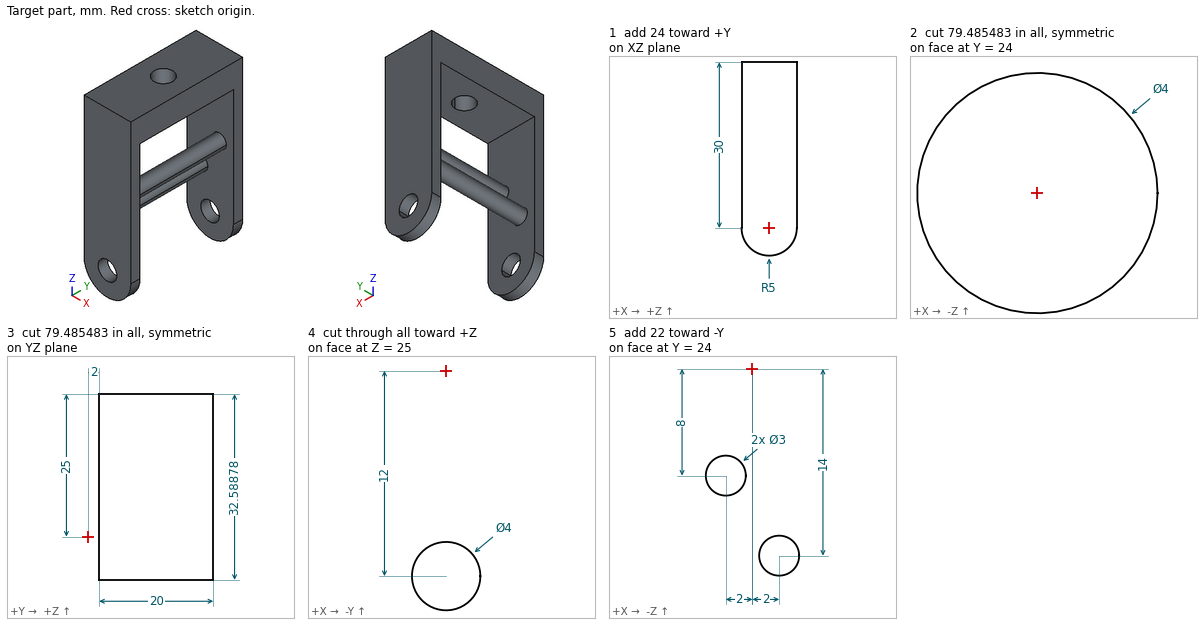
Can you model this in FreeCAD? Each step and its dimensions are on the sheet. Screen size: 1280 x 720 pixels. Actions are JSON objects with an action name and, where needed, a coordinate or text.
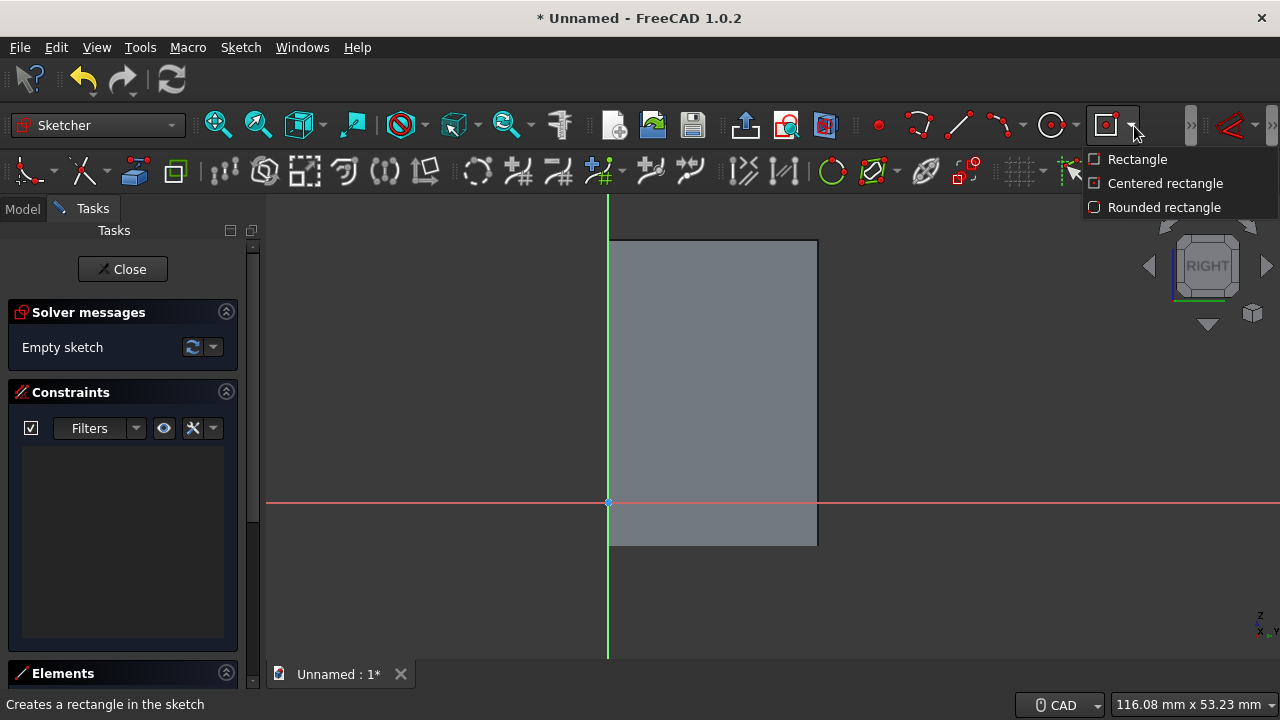
{"action": "left_click", "coordinate": [1180, 159]}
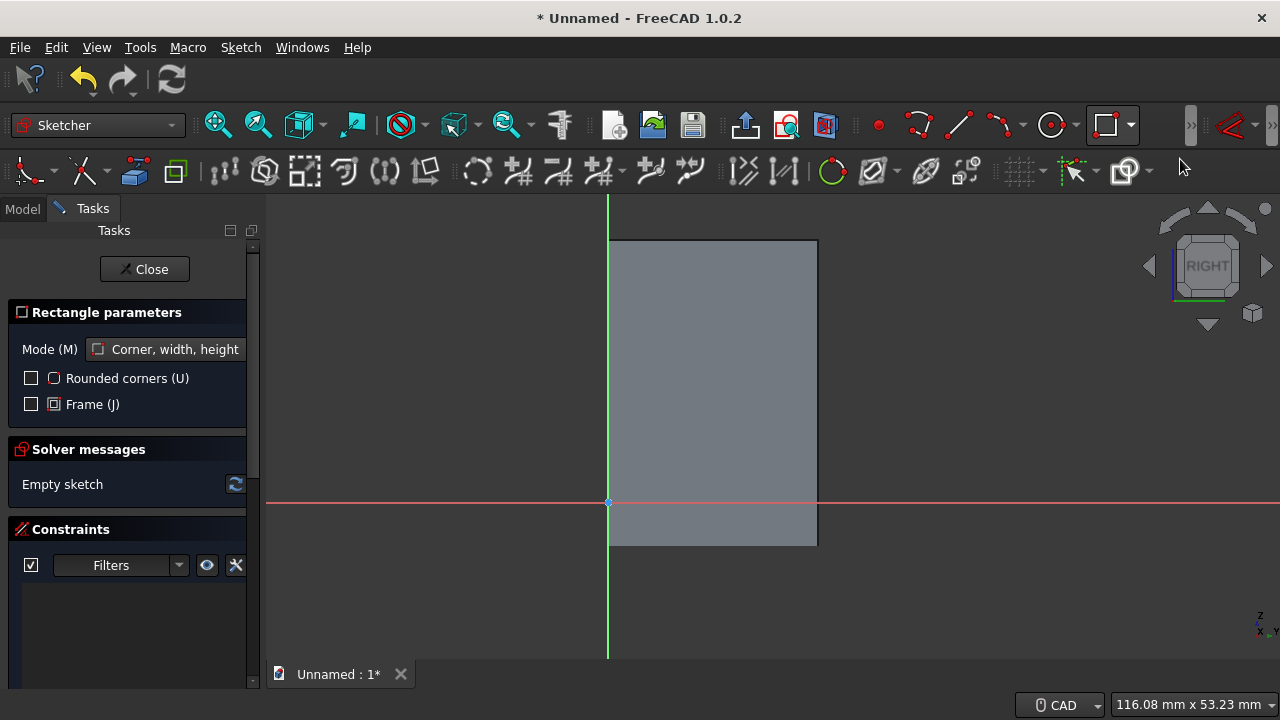
{"action": "left_click", "coordinate": [626, 284]}
{"action": "mouse_move", "coordinate": [801, 569]}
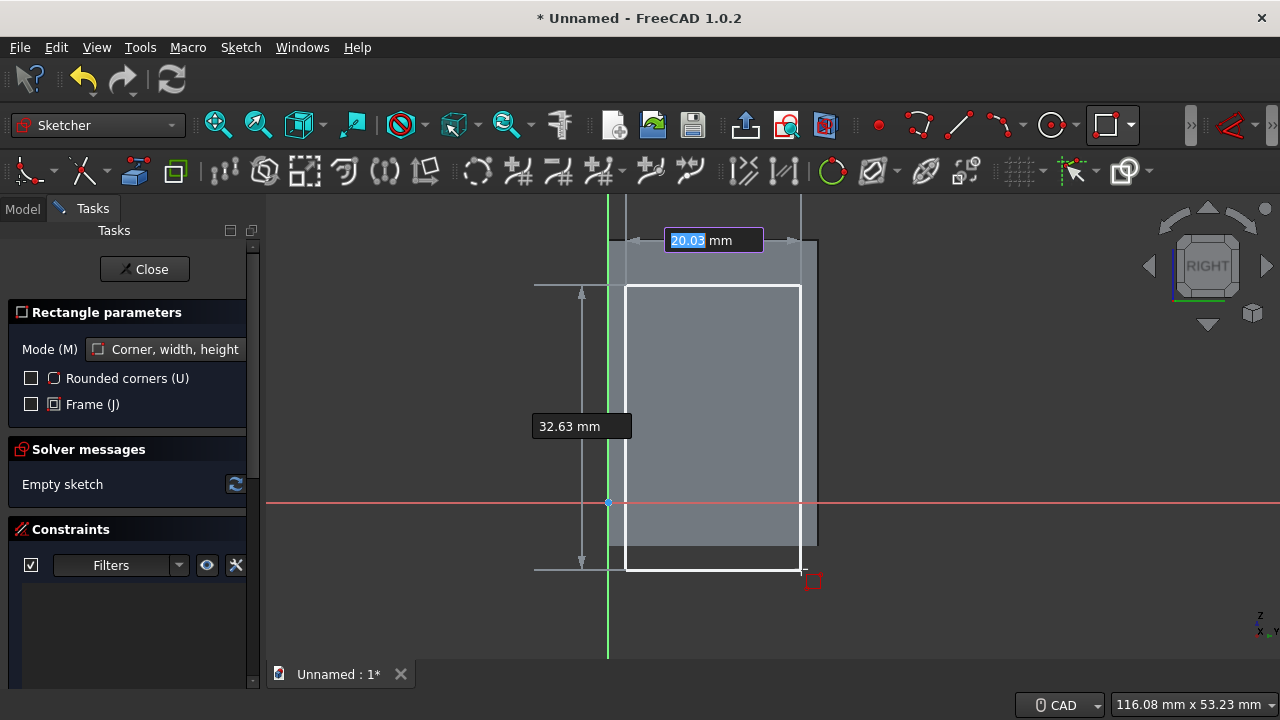
{"action": "type", "text": "20"}
{"action": "key", "text": "Tab"}
{"action": "type", "text": "32.58878"}
{"action": "key", "text": "Return"}
{"action": "key", "text": "Escape"}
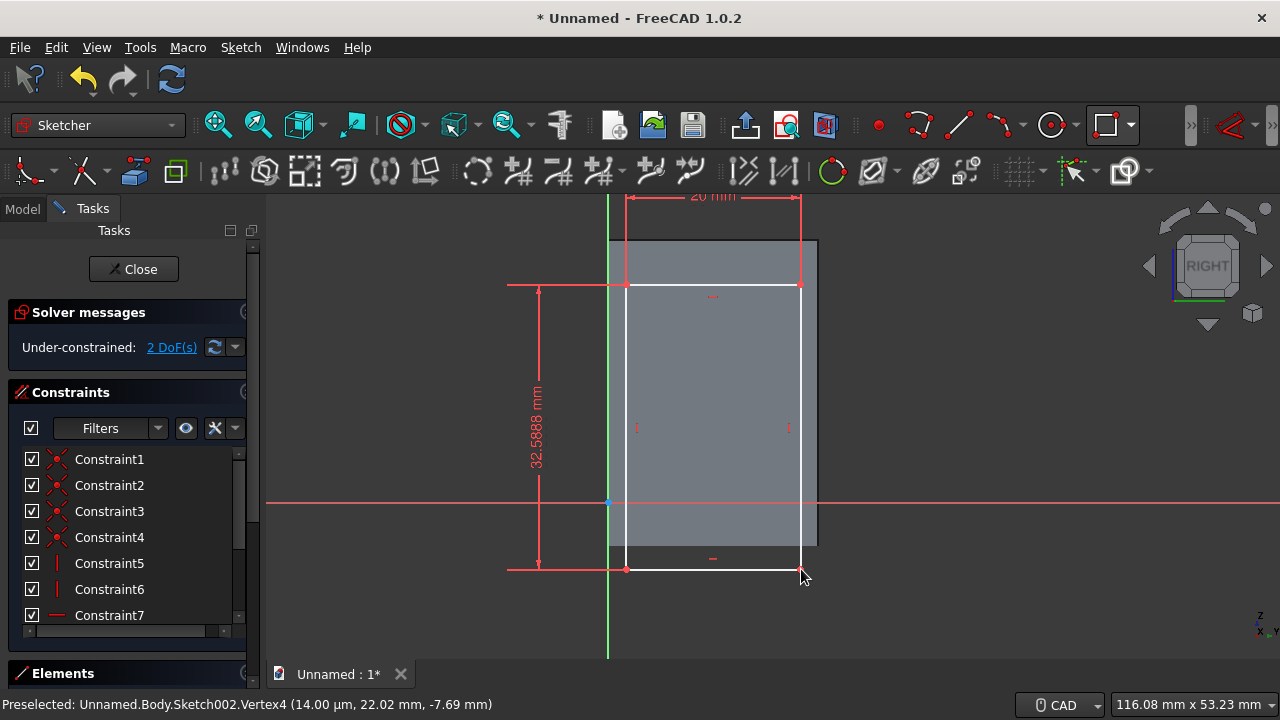
{"action": "left_click", "coordinate": [1230, 126]}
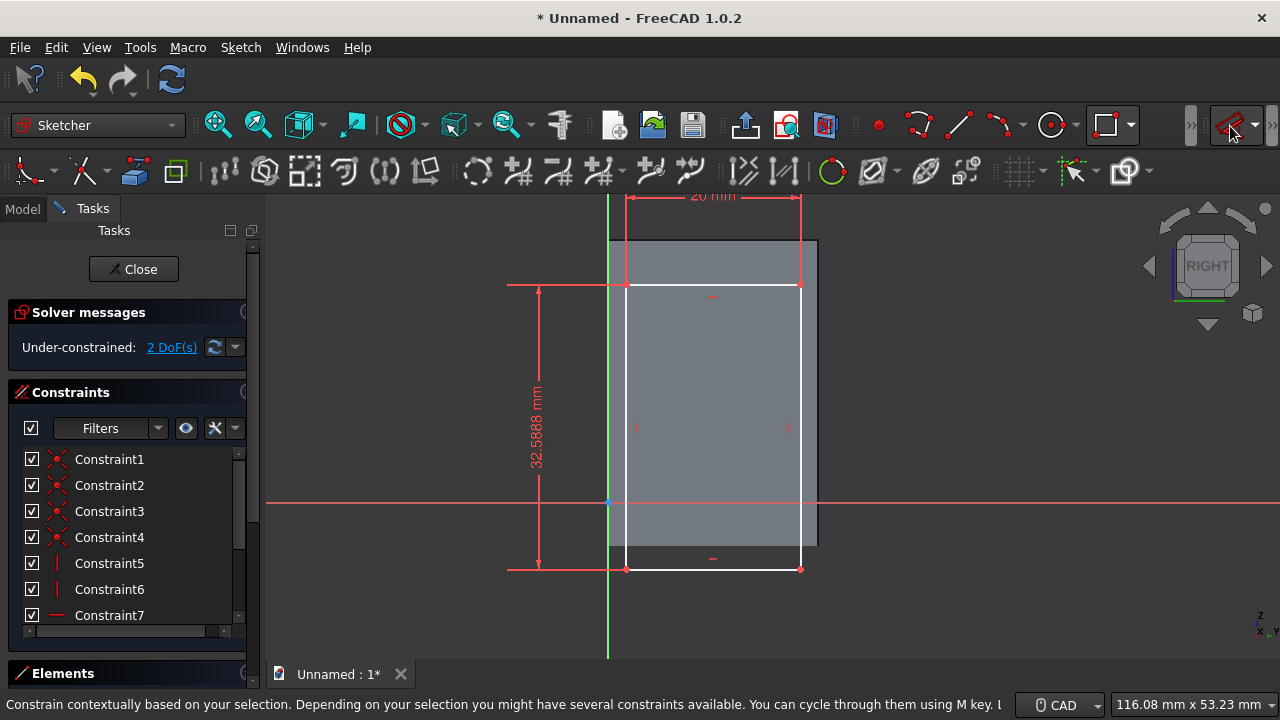
{"action": "scroll", "coordinate": [626, 285], "scroll_direction": "up", "scroll_amount": 5}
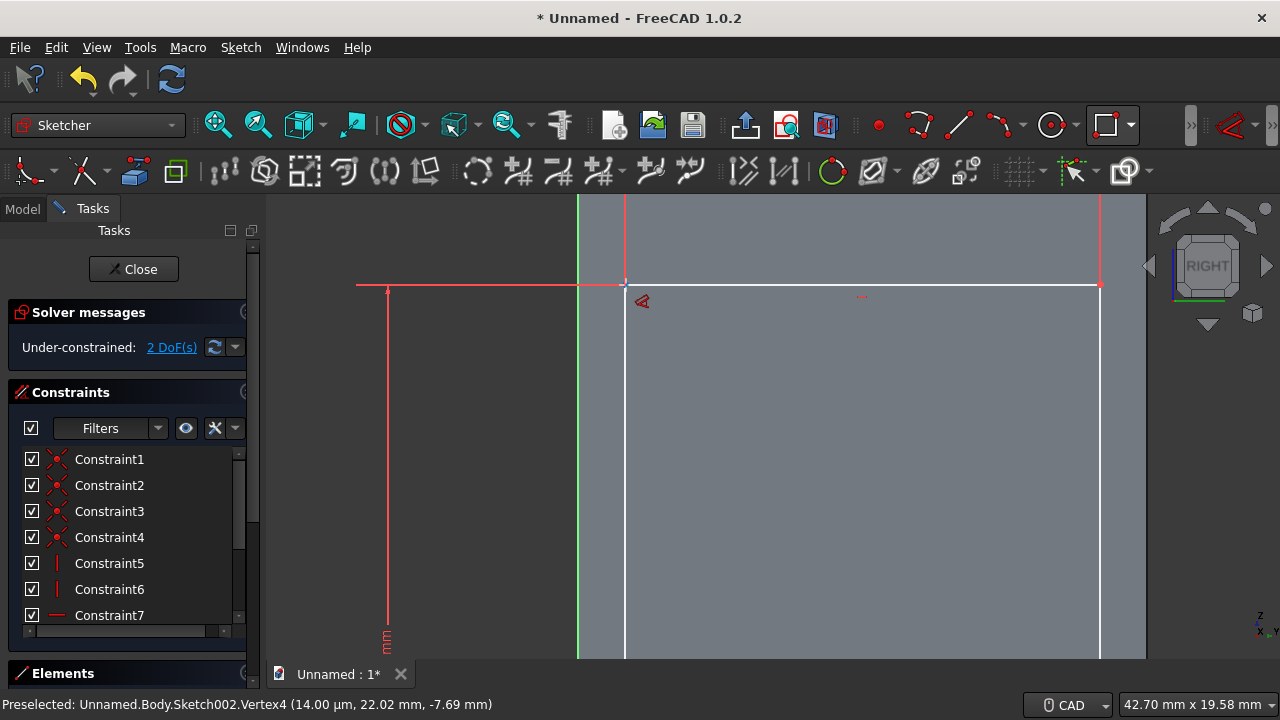
{"action": "left_click", "coordinate": [625, 285]}
{"action": "left_click", "coordinate": [601, 251]}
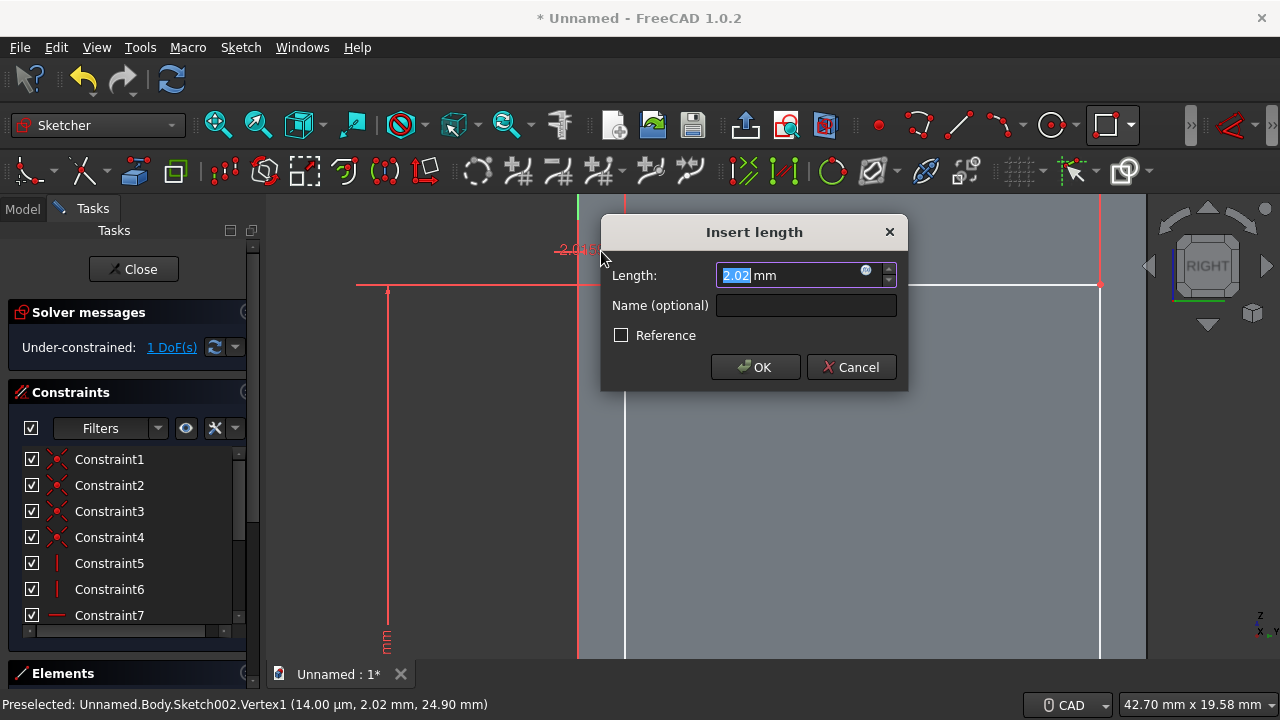
{"action": "type", "text": "2"}
{"action": "key", "text": "Return"}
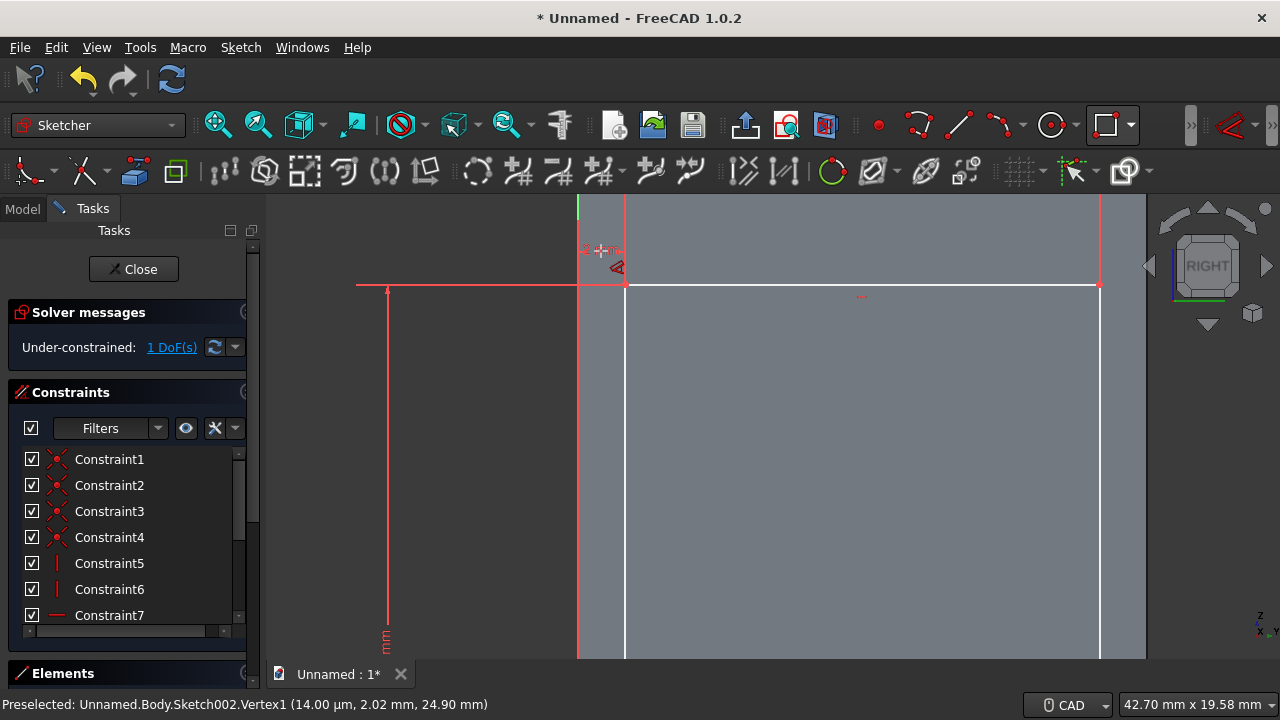
{"action": "left_click", "coordinate": [625, 285]}
{"action": "left_click", "coordinate": [544, 458]}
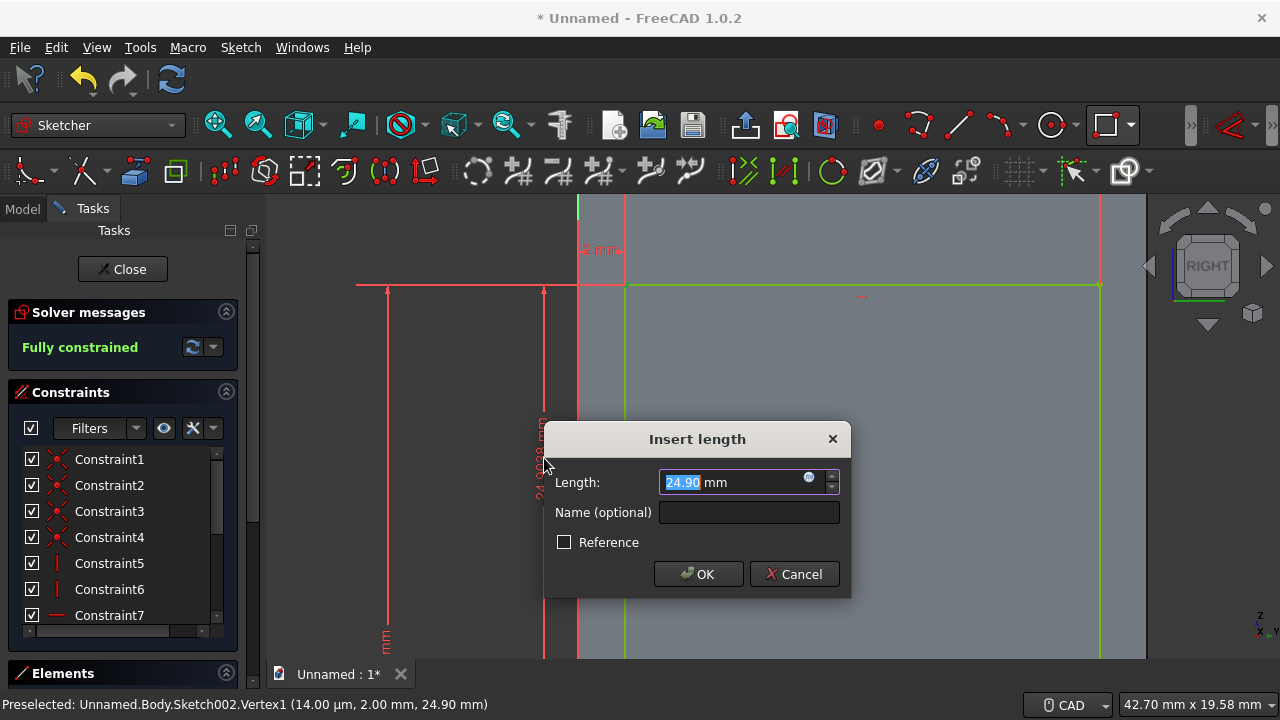
{"action": "type", "text": "25"}
{"action": "key", "text": "Return"}
{"action": "key", "text": "Escape"}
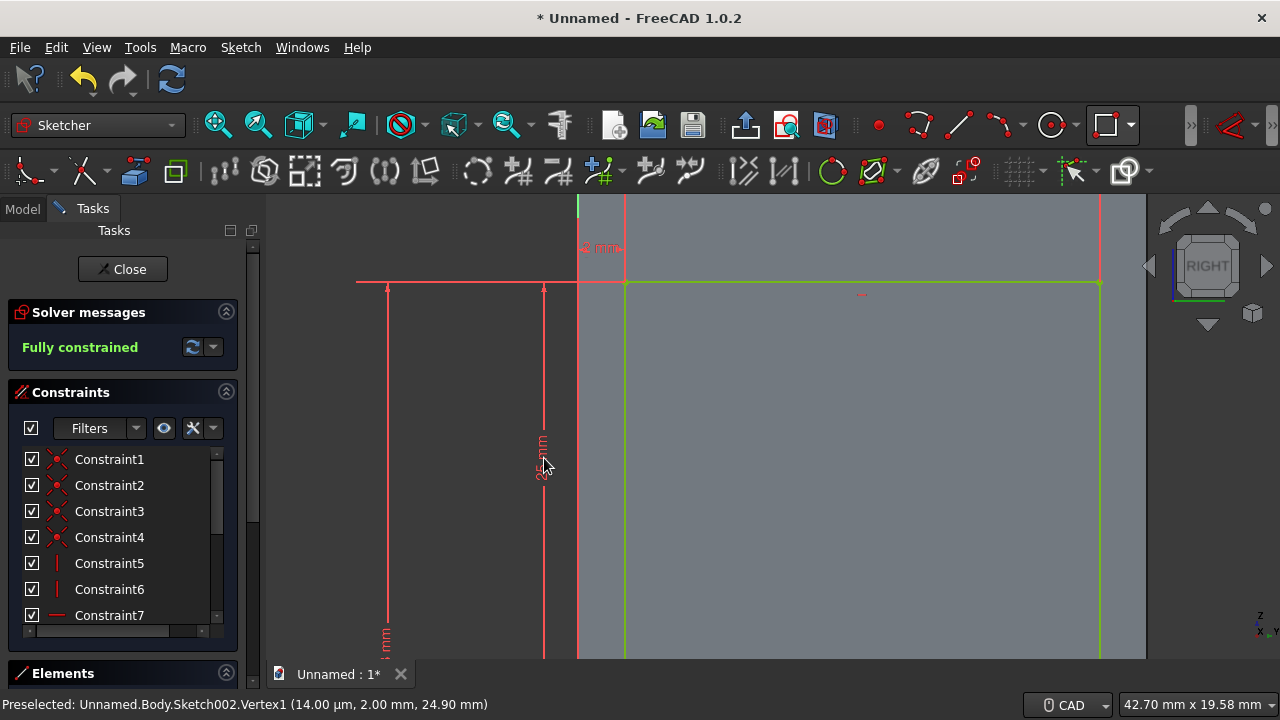
{"action": "left_click", "coordinate": [123, 269]}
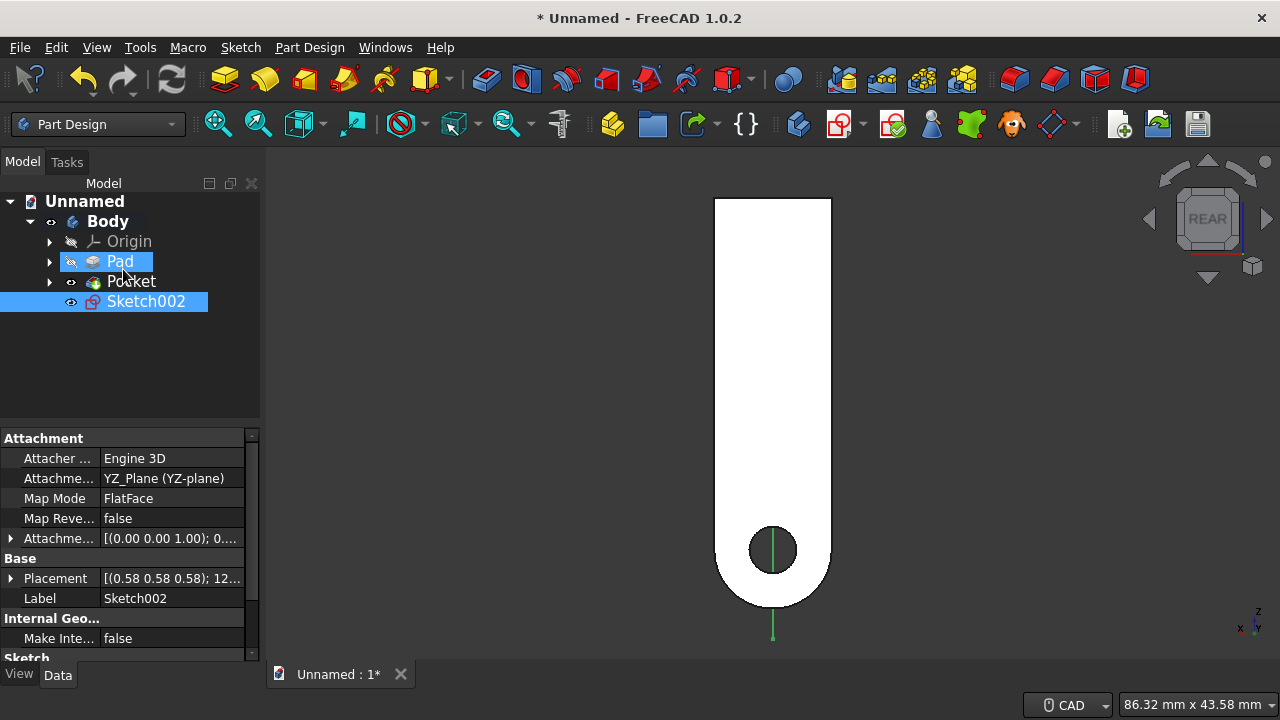
{"action": "left_click", "coordinate": [488, 80]}